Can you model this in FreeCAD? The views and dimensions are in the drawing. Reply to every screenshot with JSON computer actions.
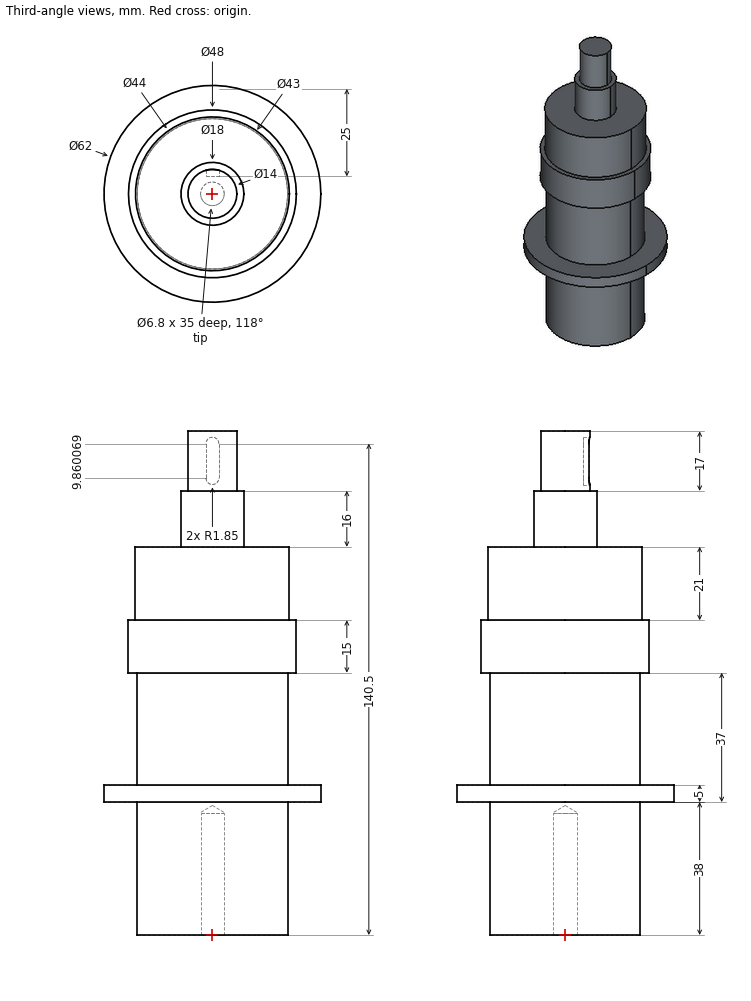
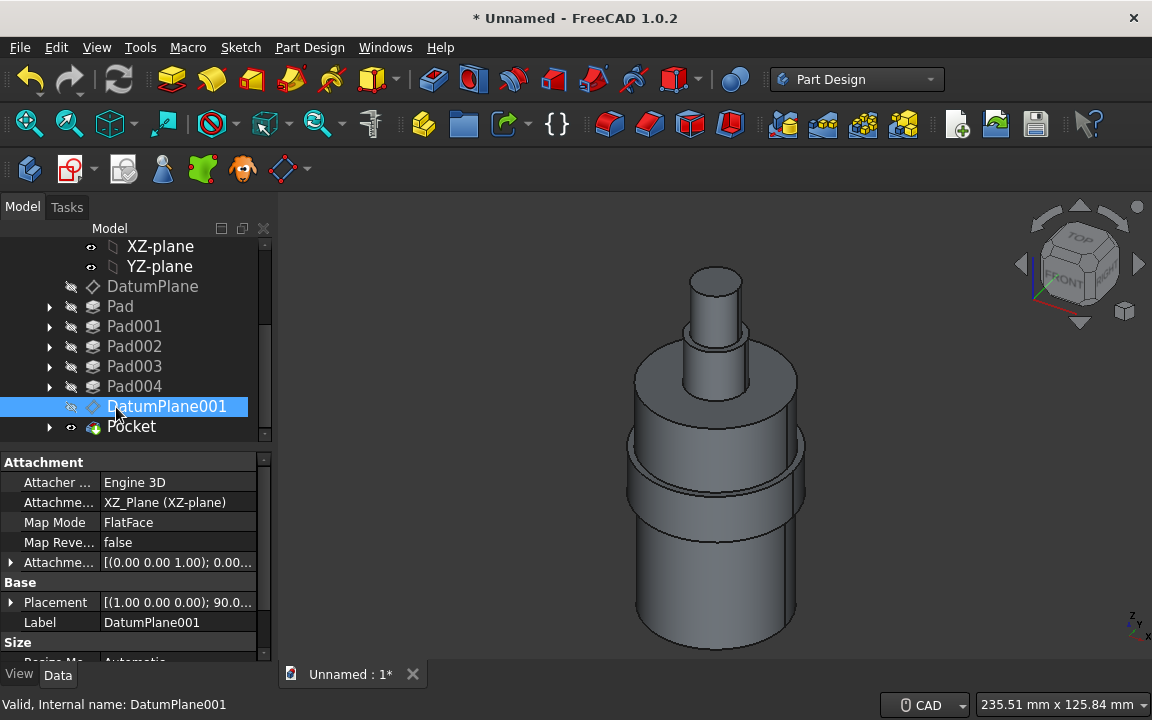
{"action": "key", "text": "v f"}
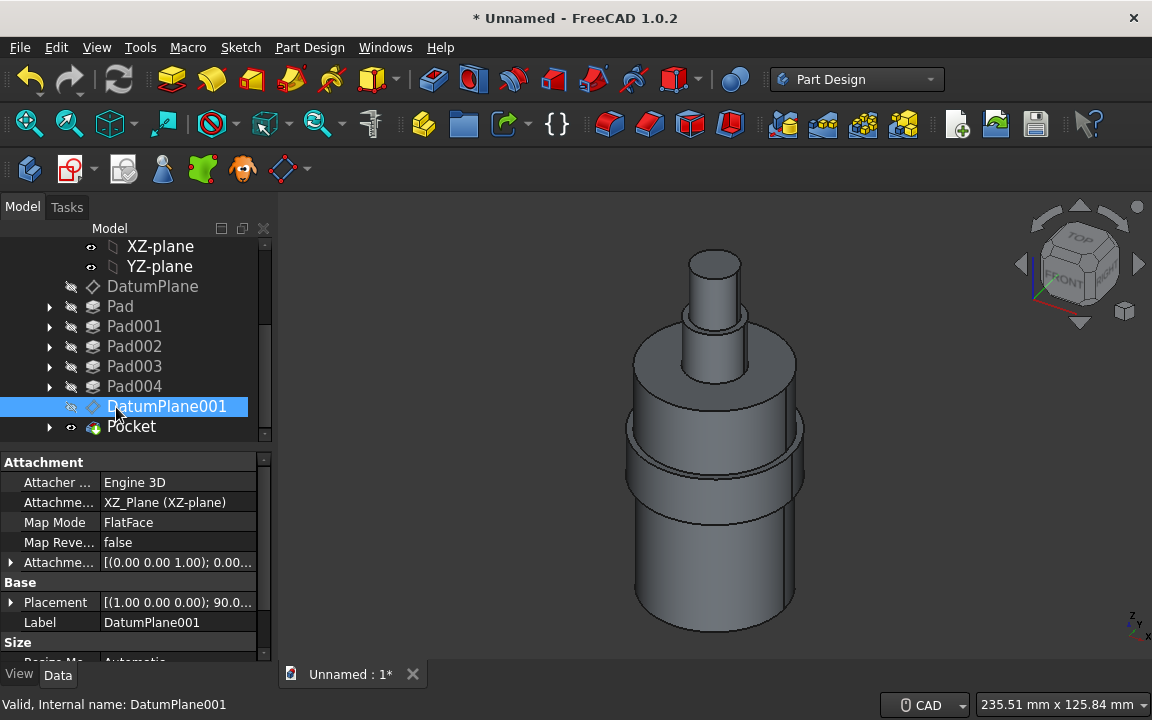
{"action": "left_click", "coordinate": [318, 619]}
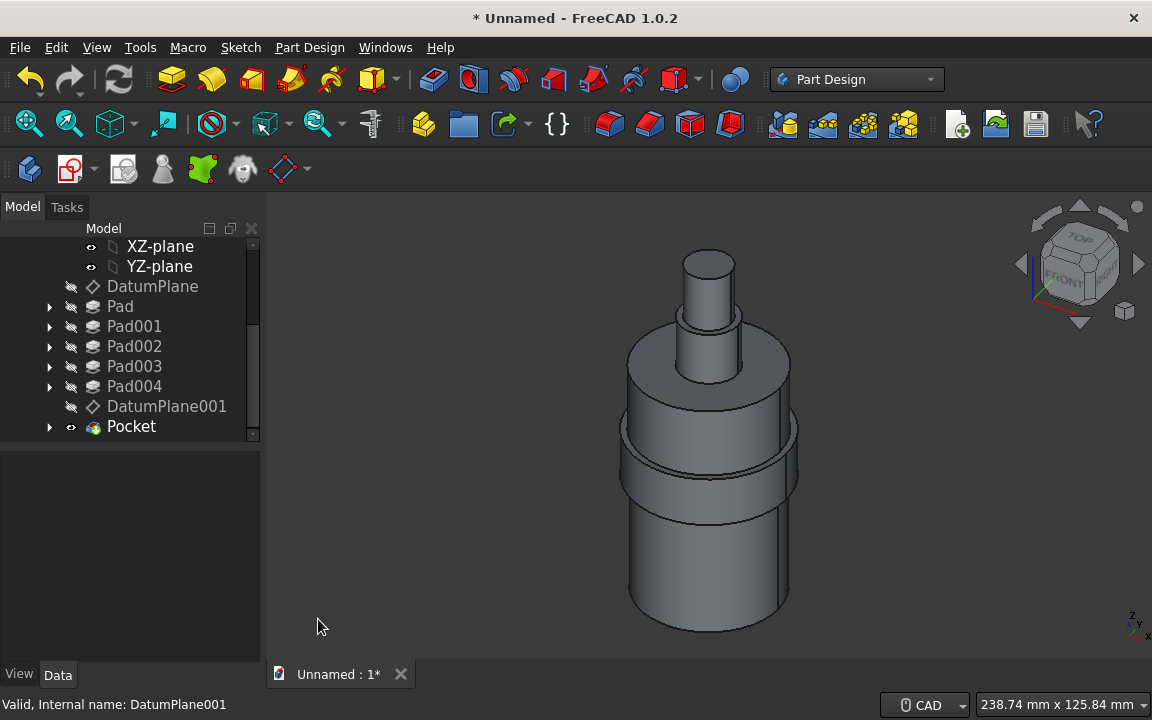
{"action": "left_click", "coordinate": [70, 170]}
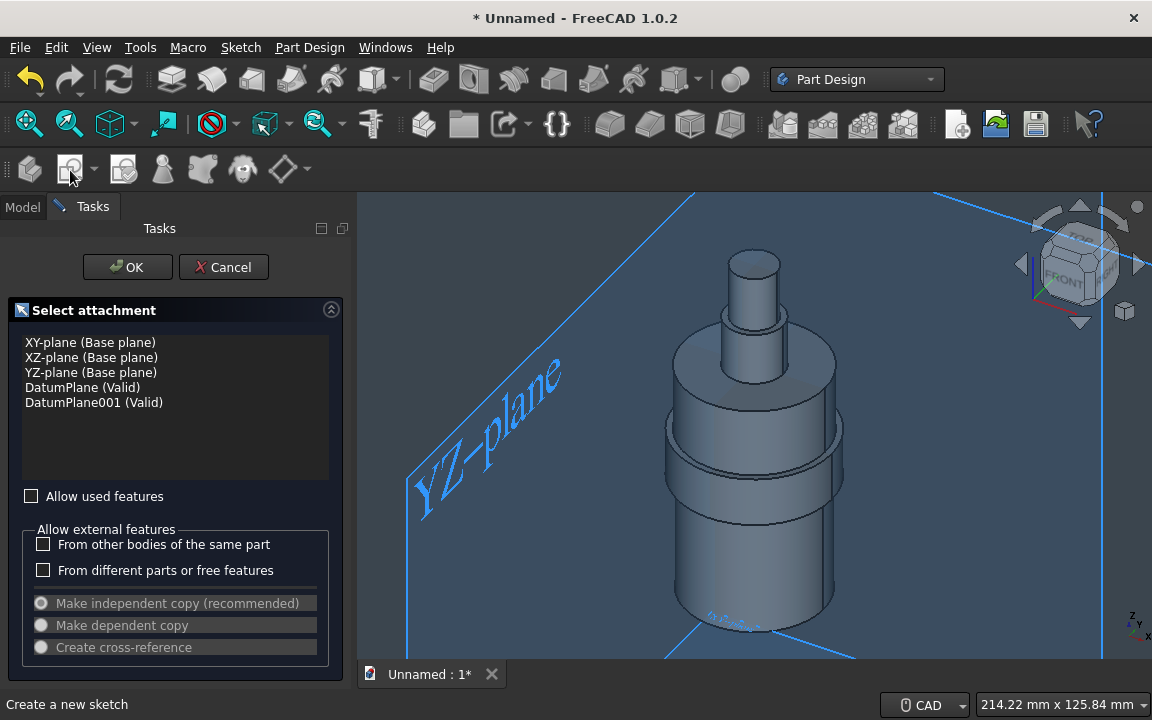
{"action": "left_click", "coordinate": [82, 342]}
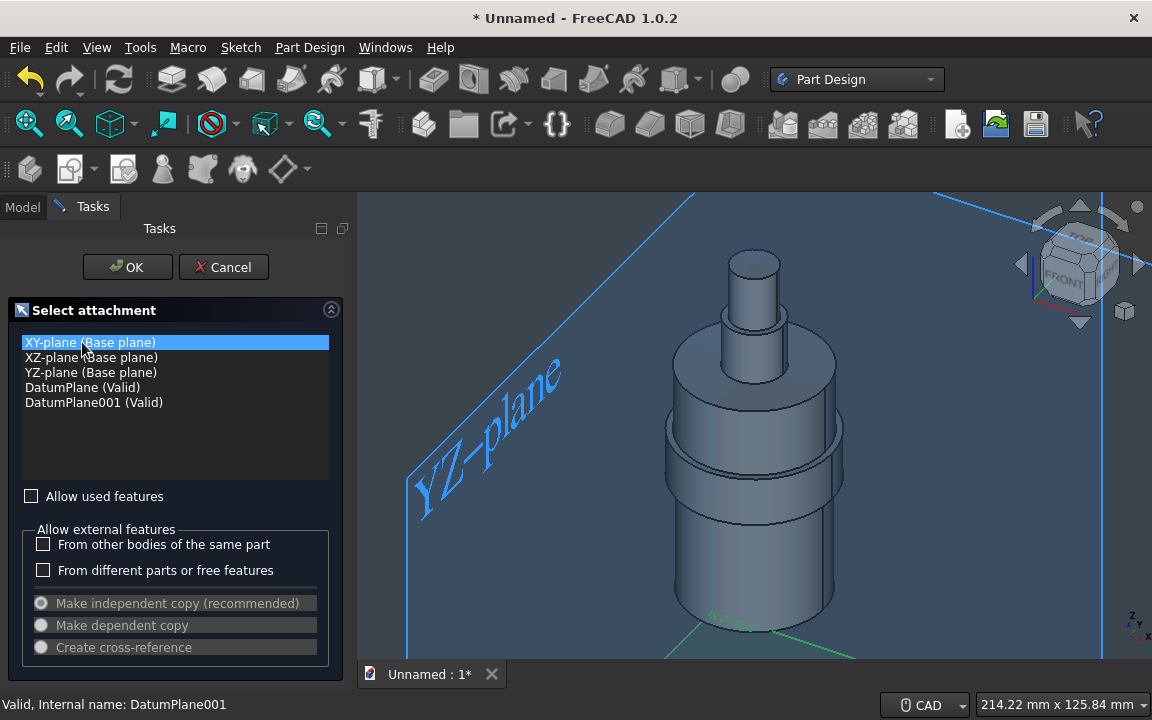
{"action": "left_click", "coordinate": [128, 267]}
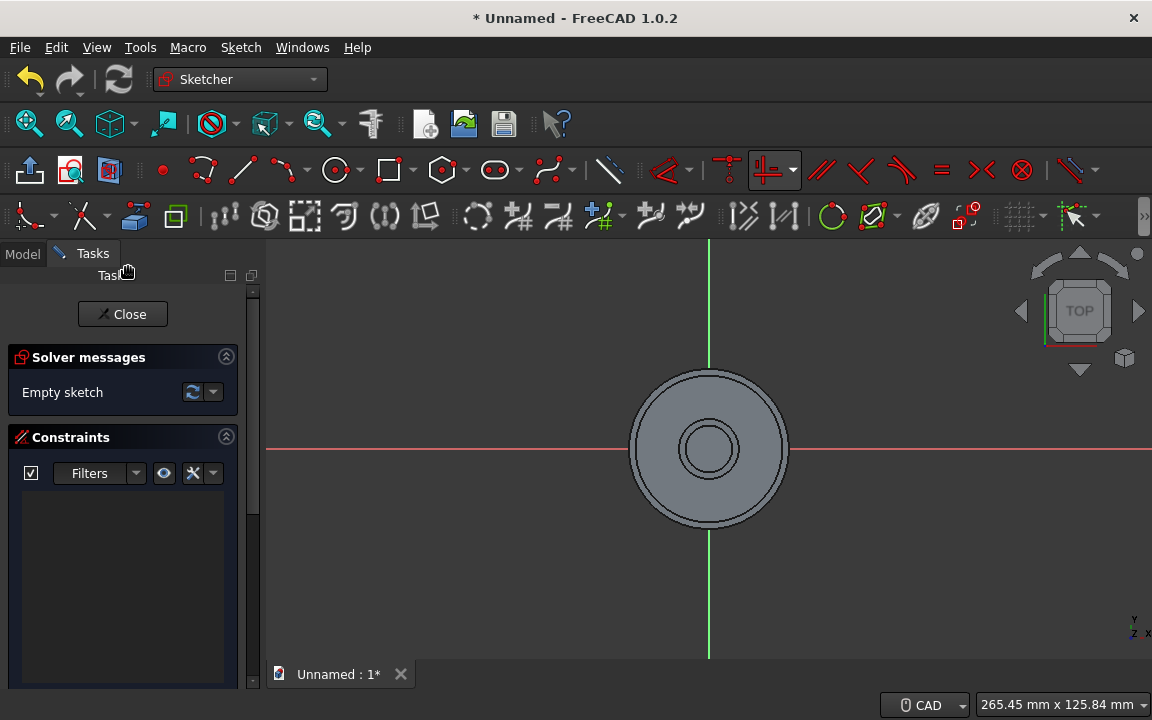
{"action": "key", "text": "q s"}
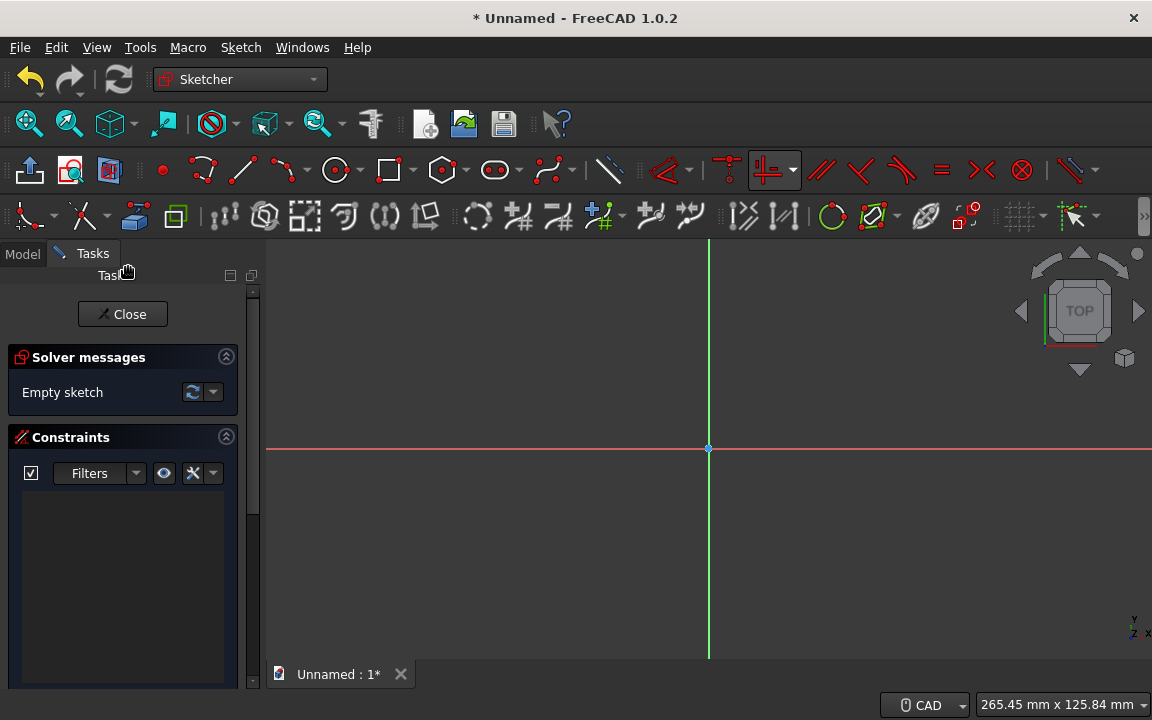
{"action": "scroll", "coordinate": [792, 449], "scroll_direction": "up", "scroll_amount": 3}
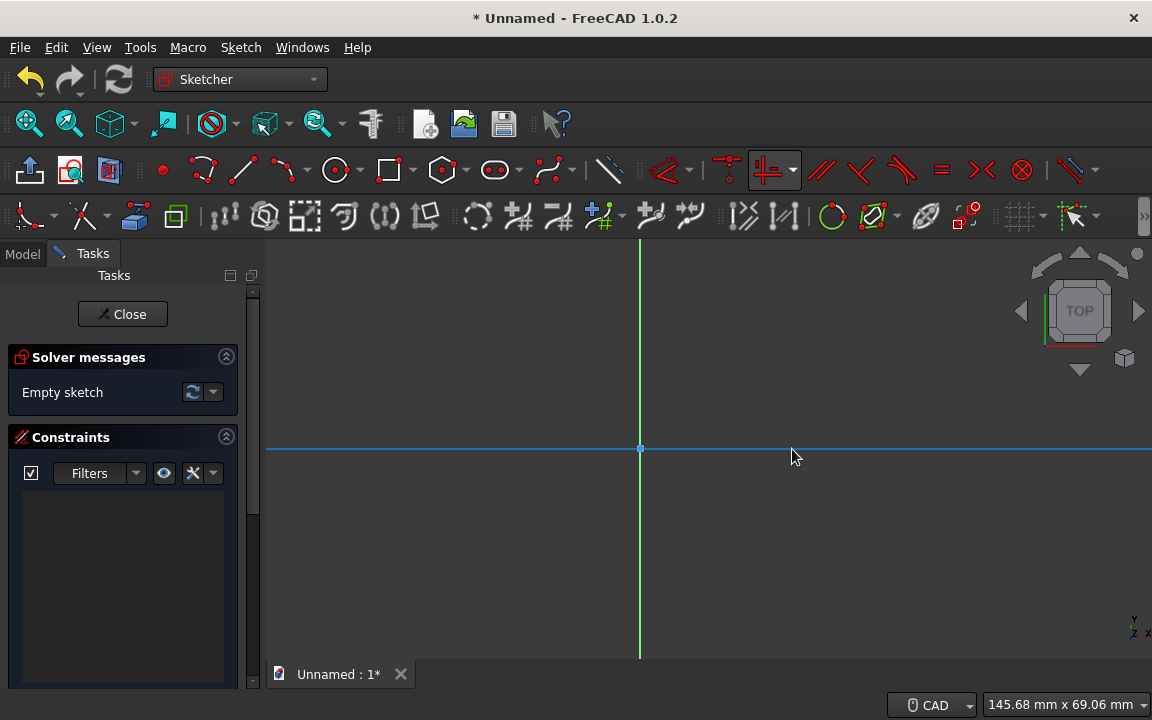
{"action": "left_click", "coordinate": [336, 170]}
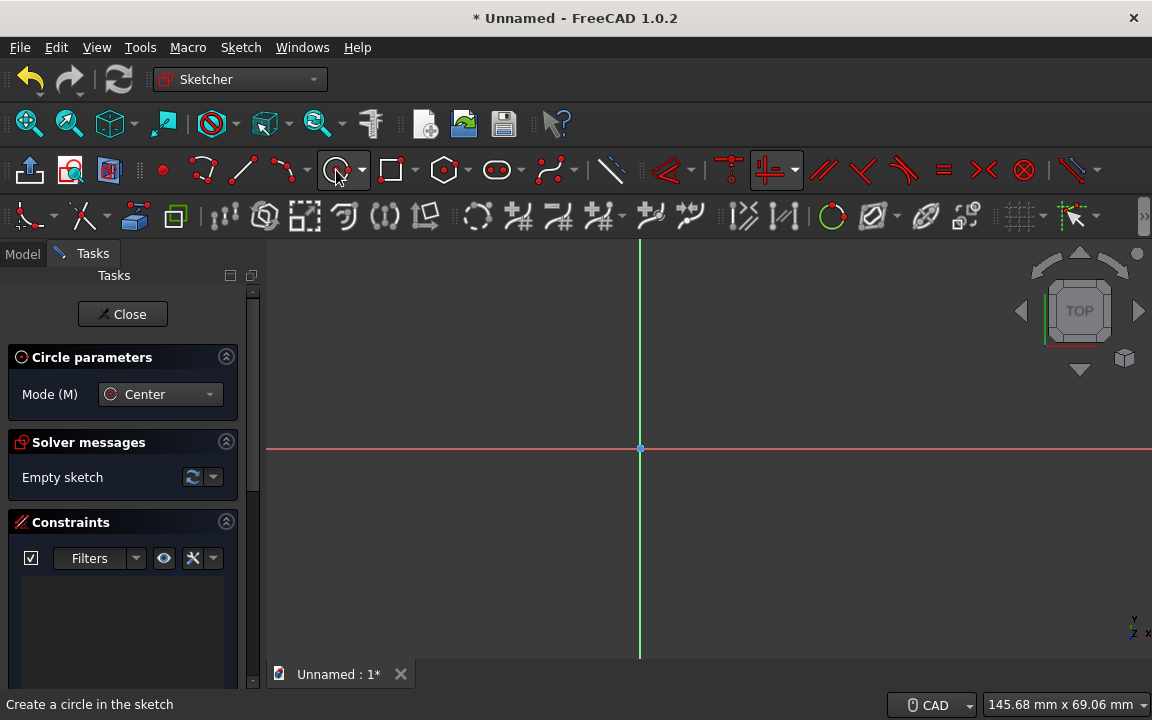
{"action": "left_click", "coordinate": [640, 449]}
{"action": "left_click", "coordinate": [733, 356]}
{"action": "key", "text": "Escape"}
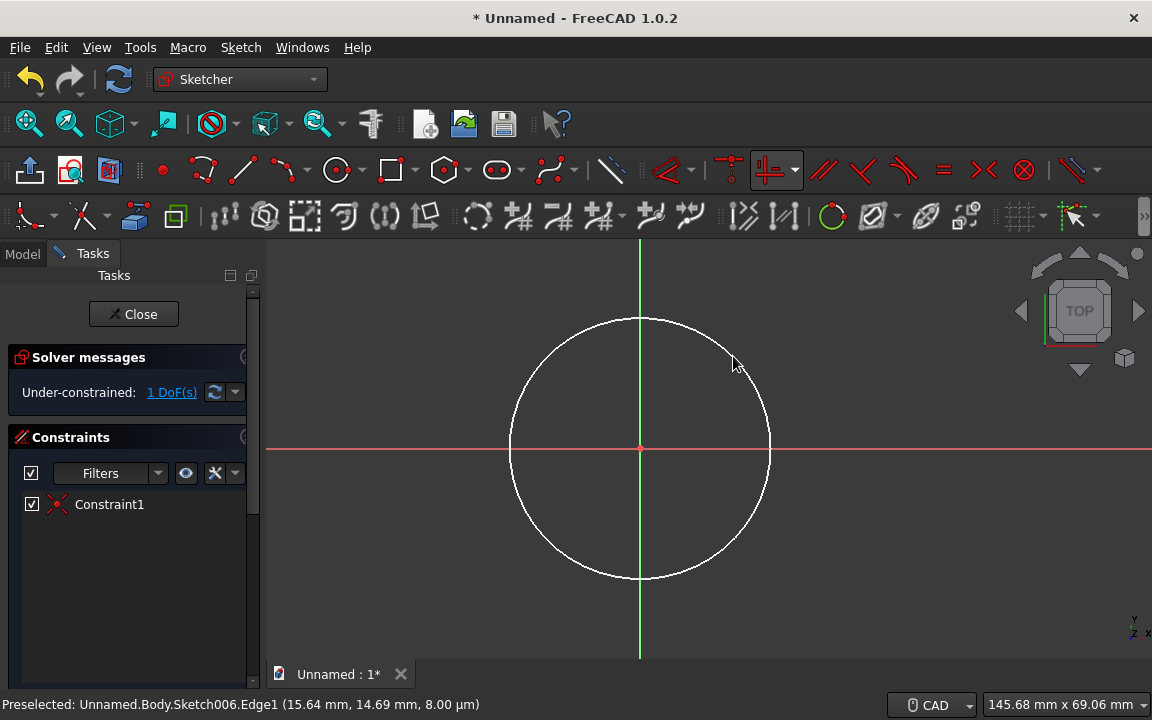
{"action": "left_click", "coordinate": [666, 170]}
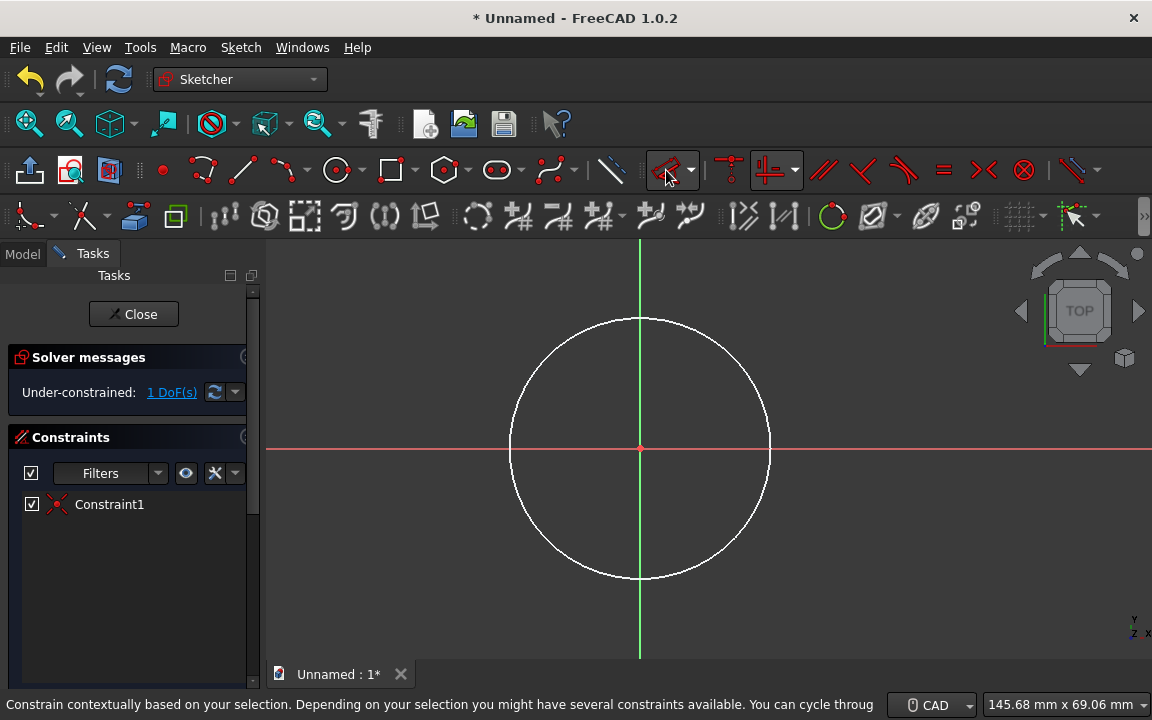
{"action": "left_click", "coordinate": [732, 356]}
{"action": "left_click", "coordinate": [755, 333]}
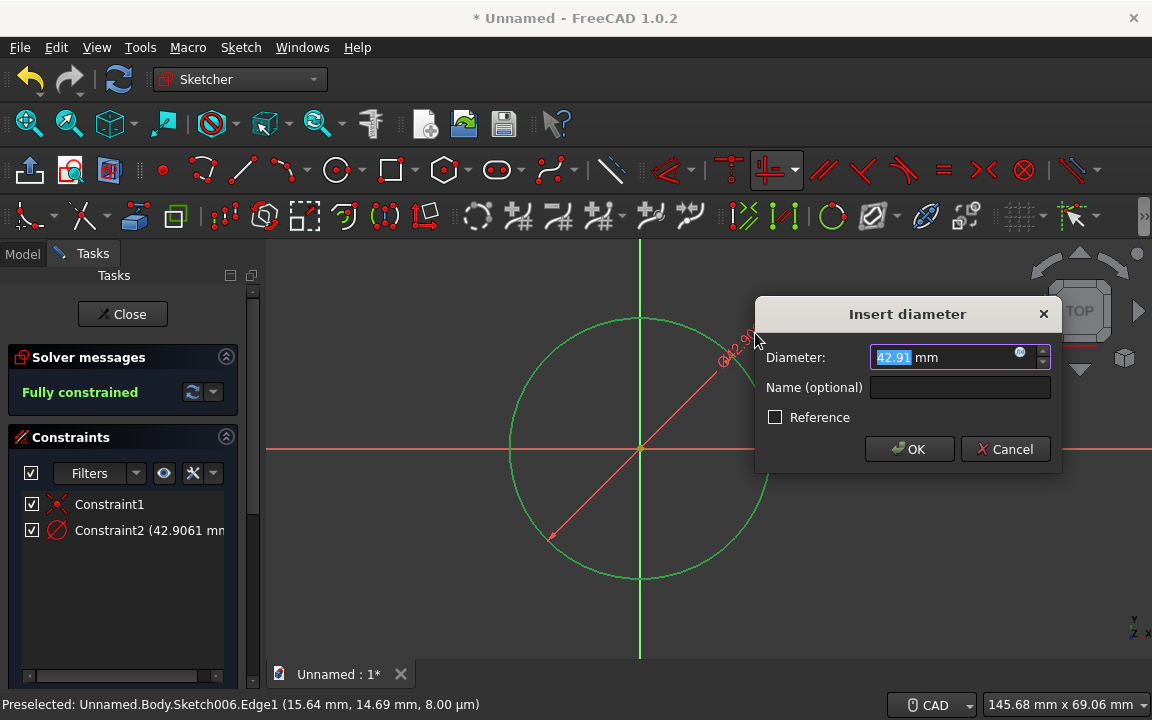
{"action": "type", "text": "43"}
{"action": "key", "text": "Return"}
{"action": "key", "text": "Escape"}